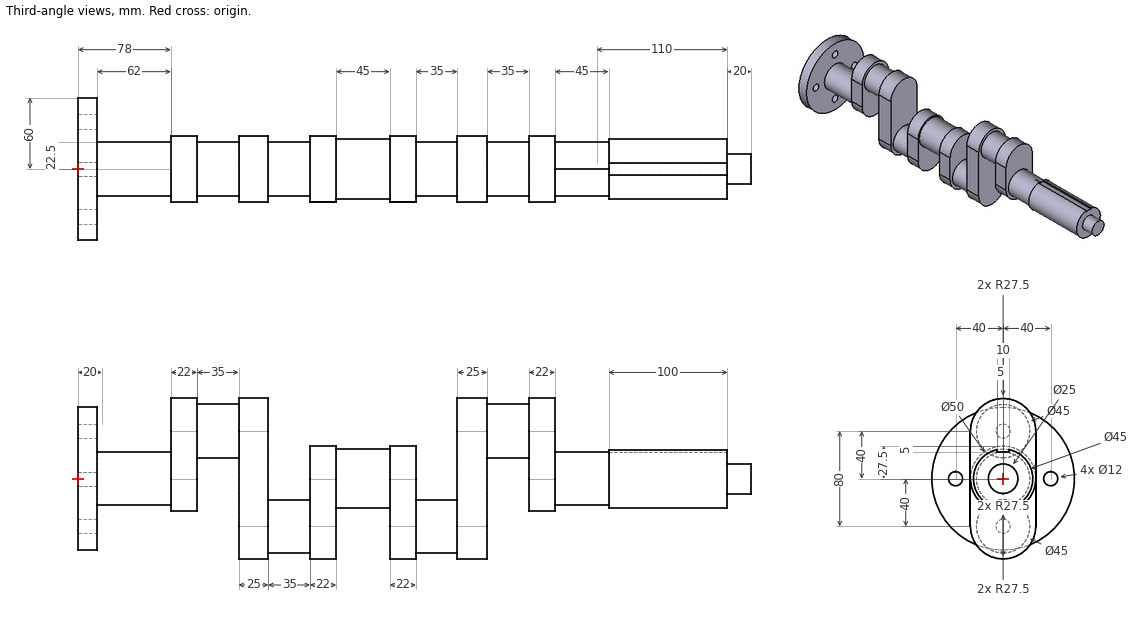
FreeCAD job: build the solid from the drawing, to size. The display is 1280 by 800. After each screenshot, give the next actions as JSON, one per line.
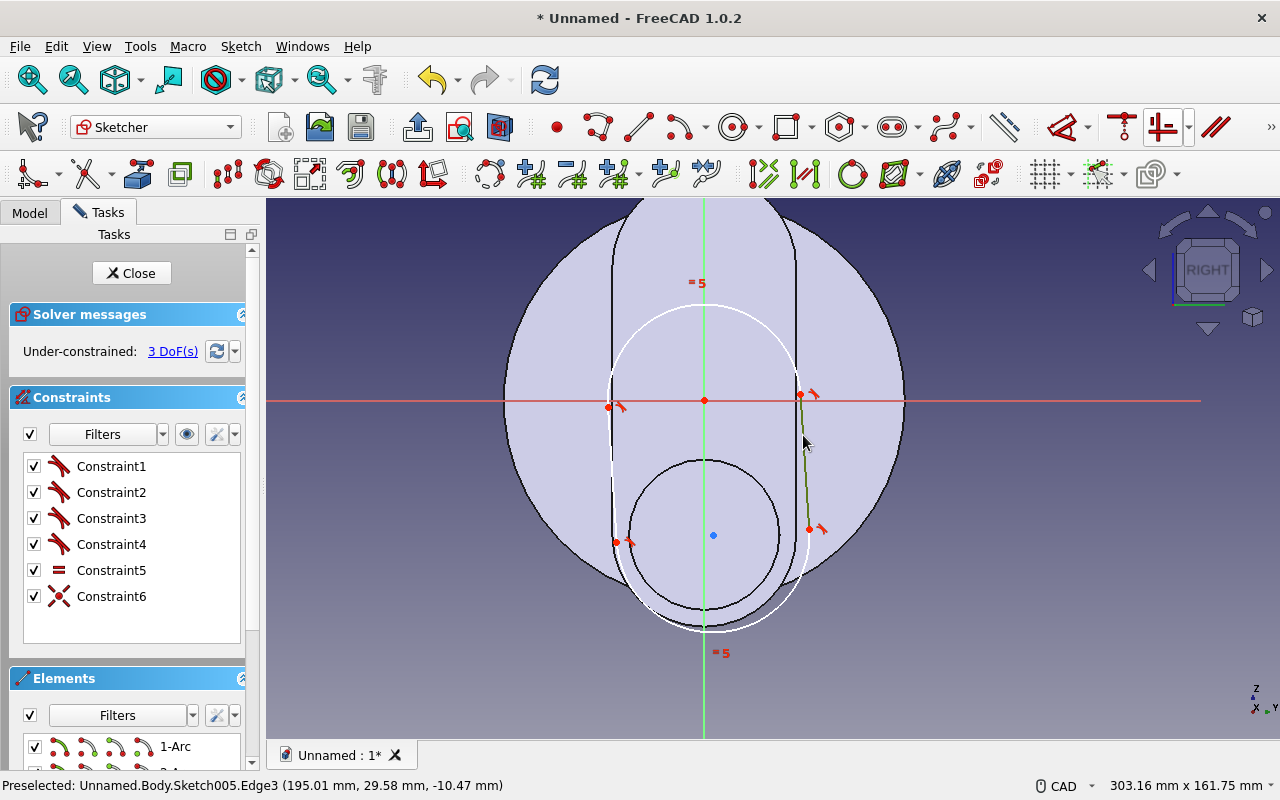
{"action": "left_click", "coordinate": [1188, 128]}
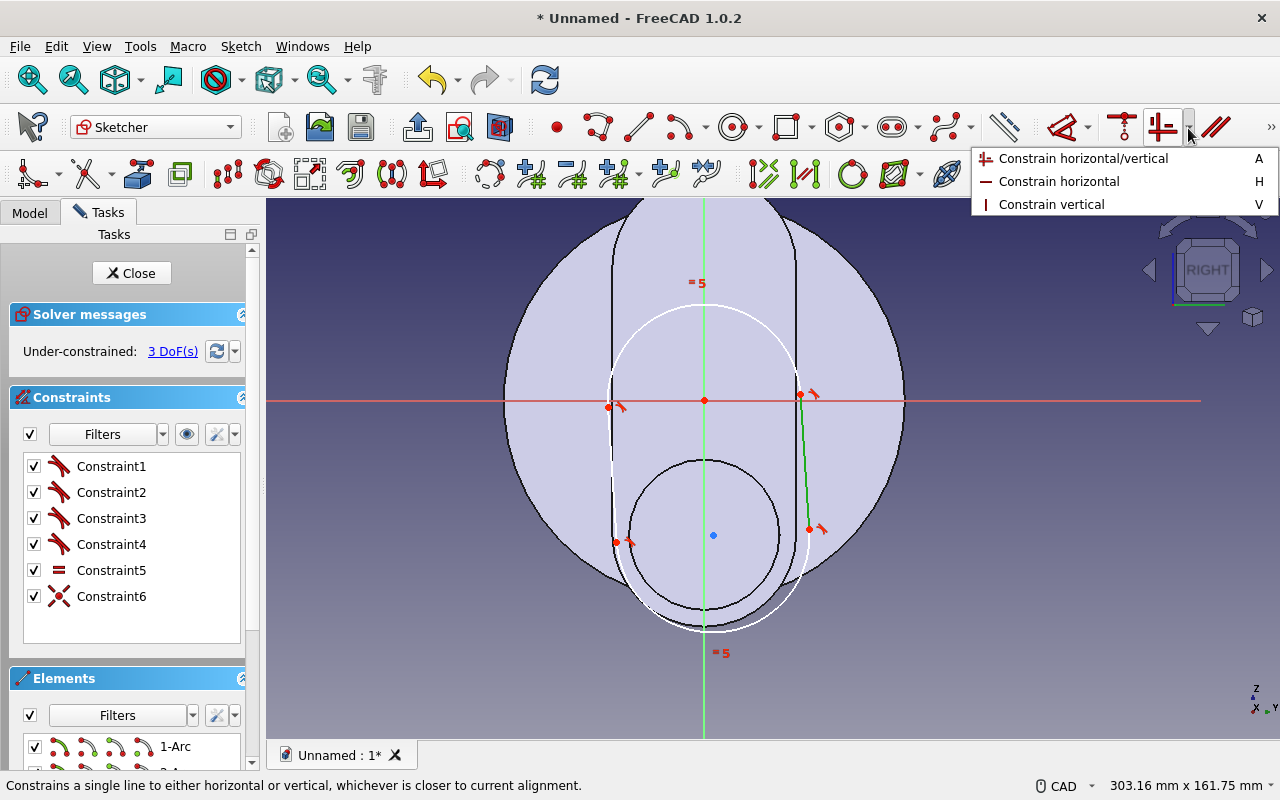
{"action": "left_click", "coordinate": [1125, 204]}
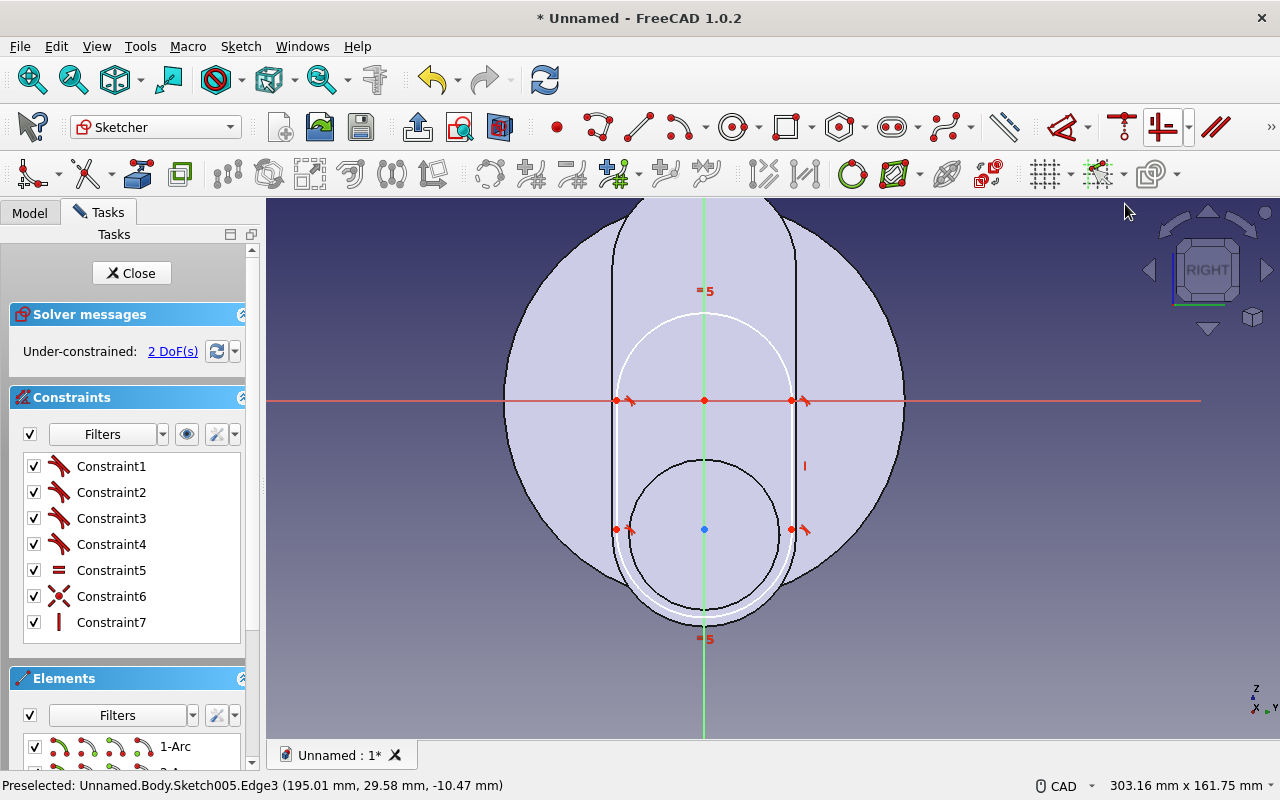
{"action": "left_click", "coordinate": [1062, 128]}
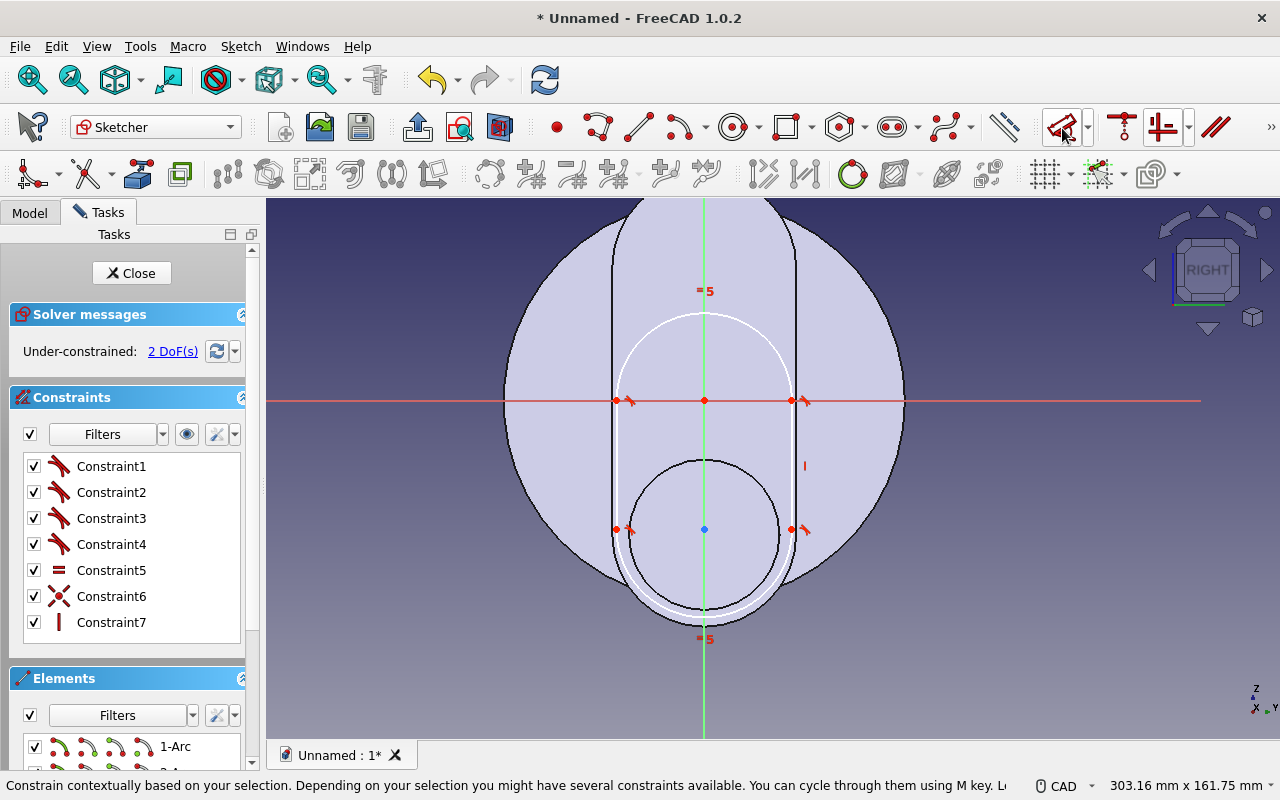
{"action": "left_click", "coordinate": [756, 330]}
{"action": "left_click", "coordinate": [775, 304]}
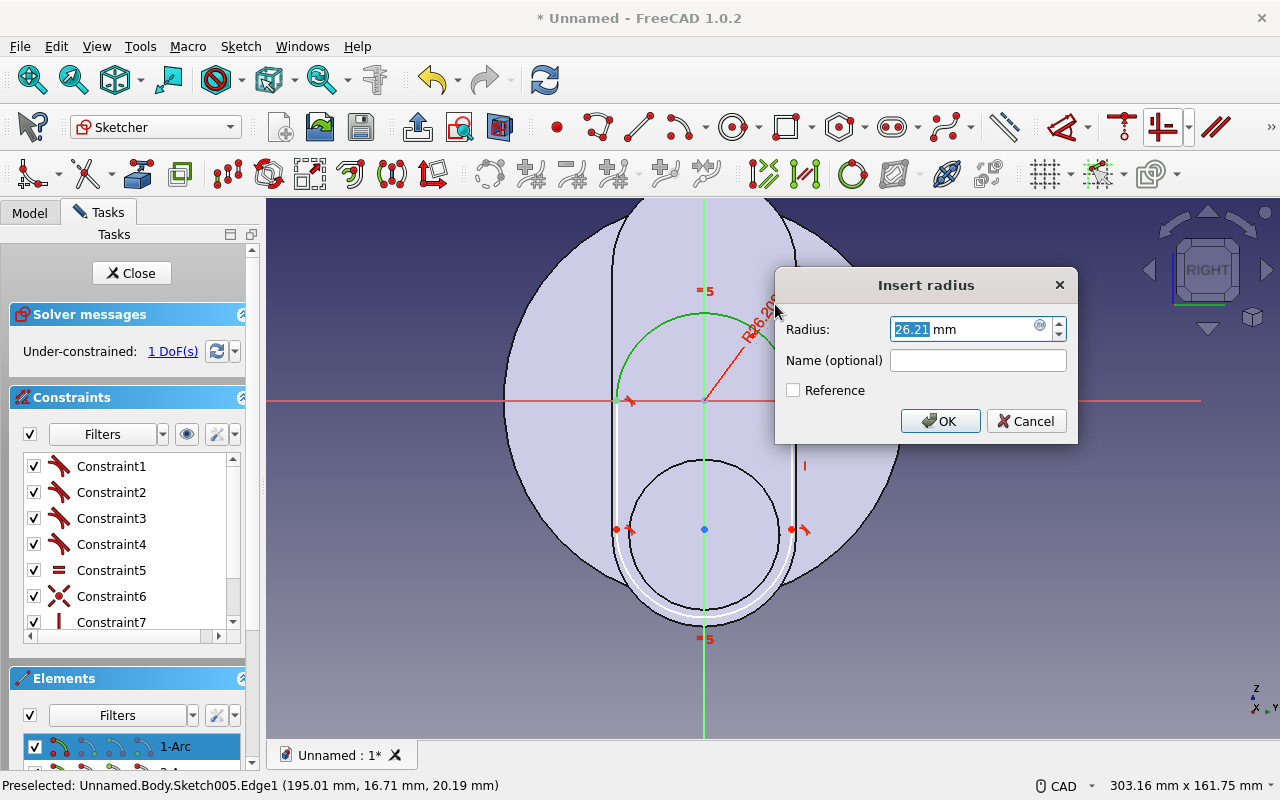
{"action": "type", "text": "27.5"}
{"action": "key", "text": "Return"}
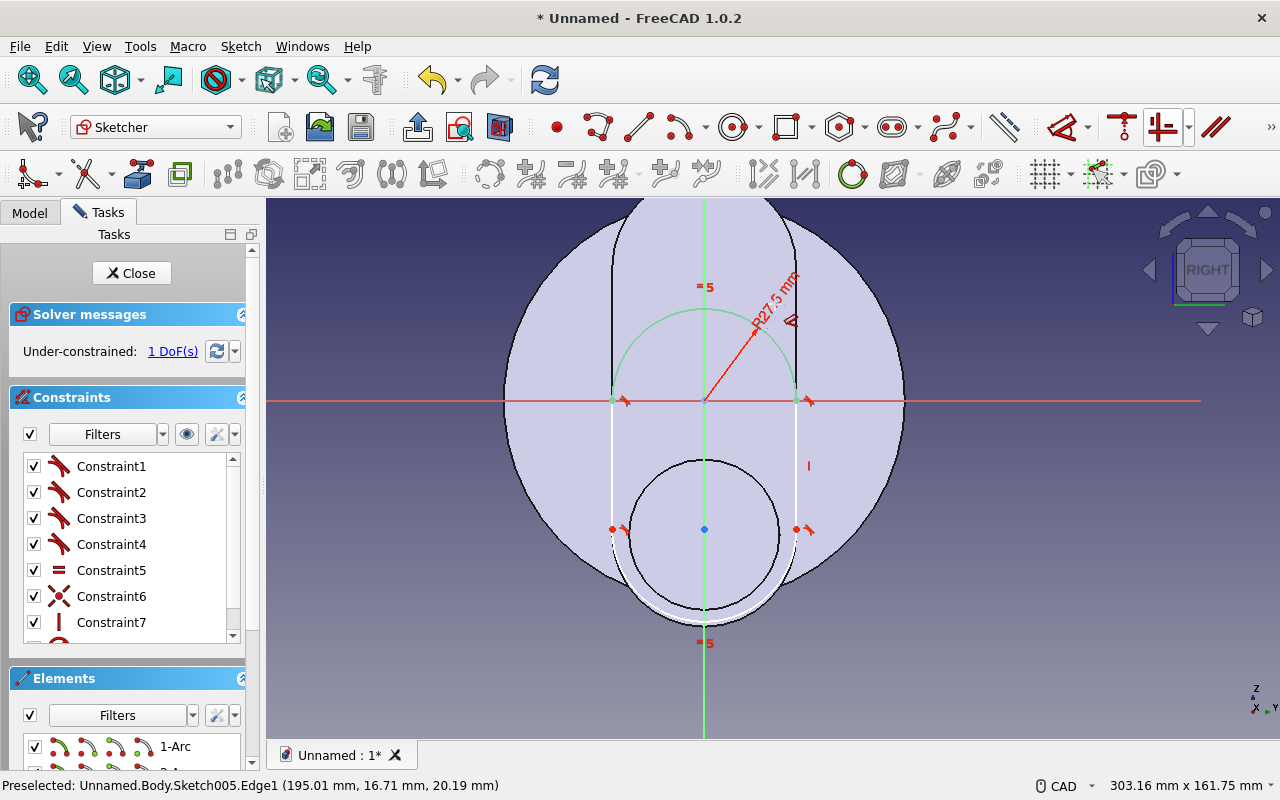
{"action": "left_click", "coordinate": [796, 440]}
{"action": "left_click", "coordinate": [830, 465]}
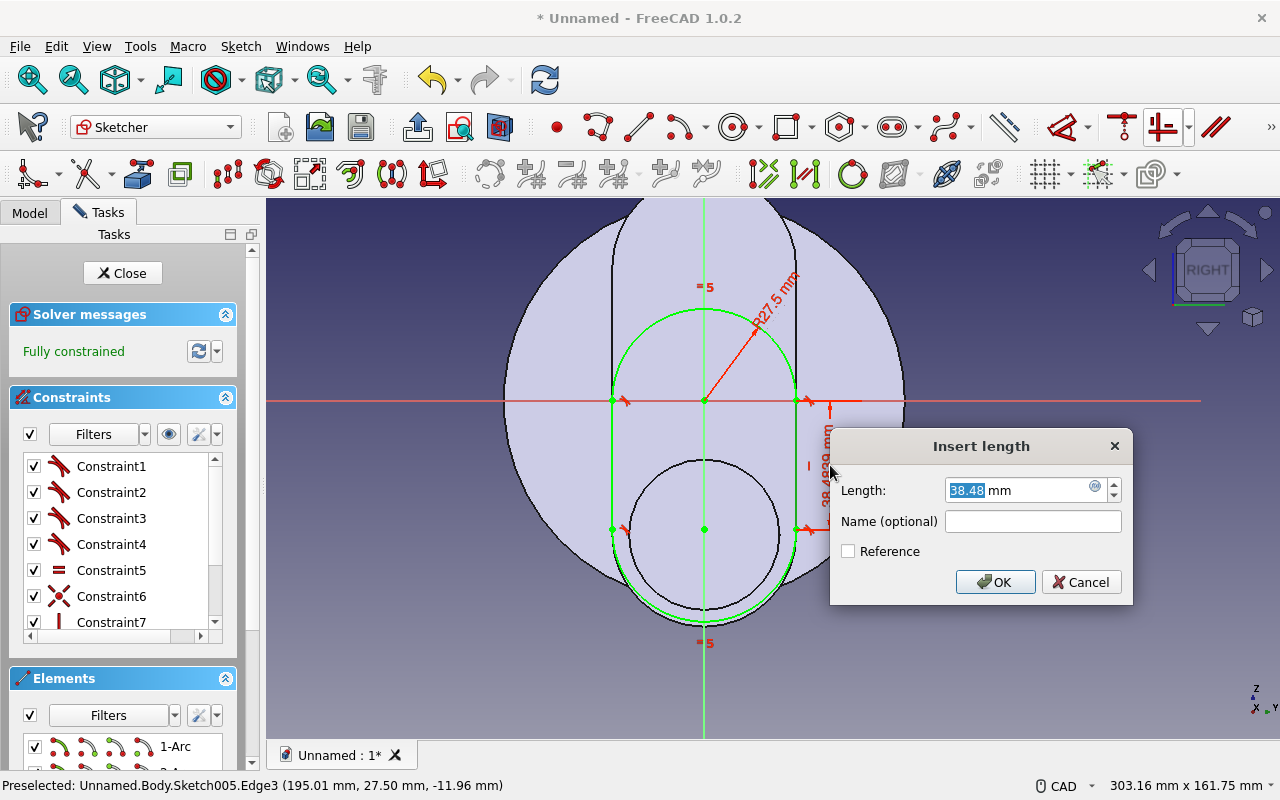
{"action": "type", "text": "40"}
{"action": "key", "text": "Return"}
{"action": "key", "text": "Escape"}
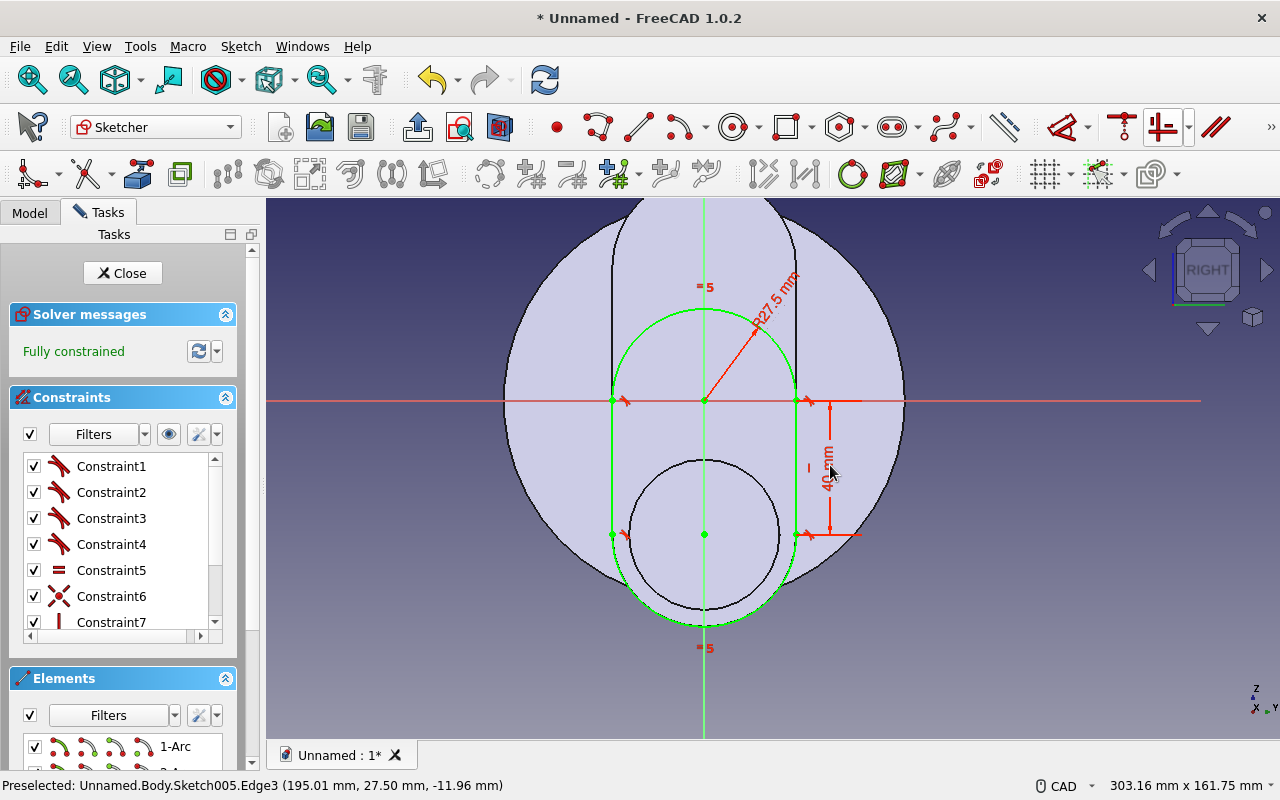
{"action": "left_click", "coordinate": [123, 273]}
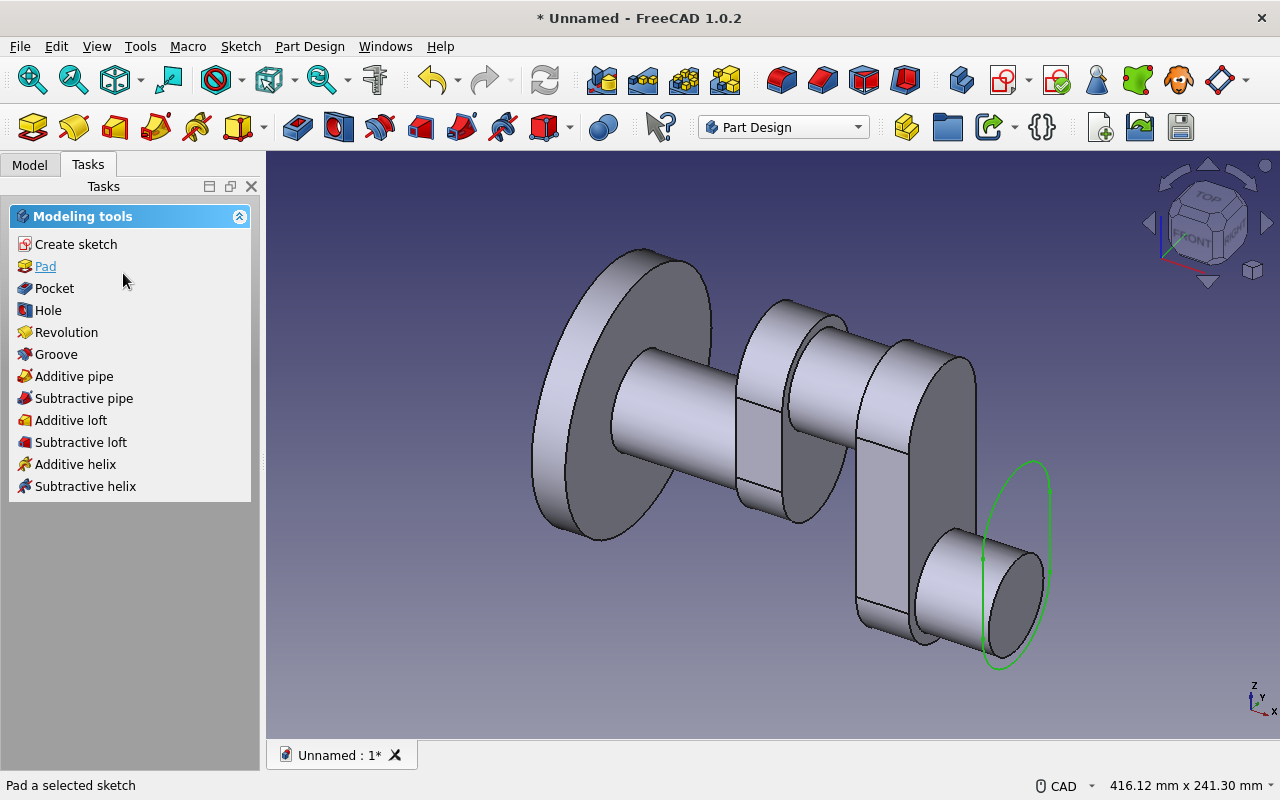
{"action": "left_click", "coordinate": [33, 128]}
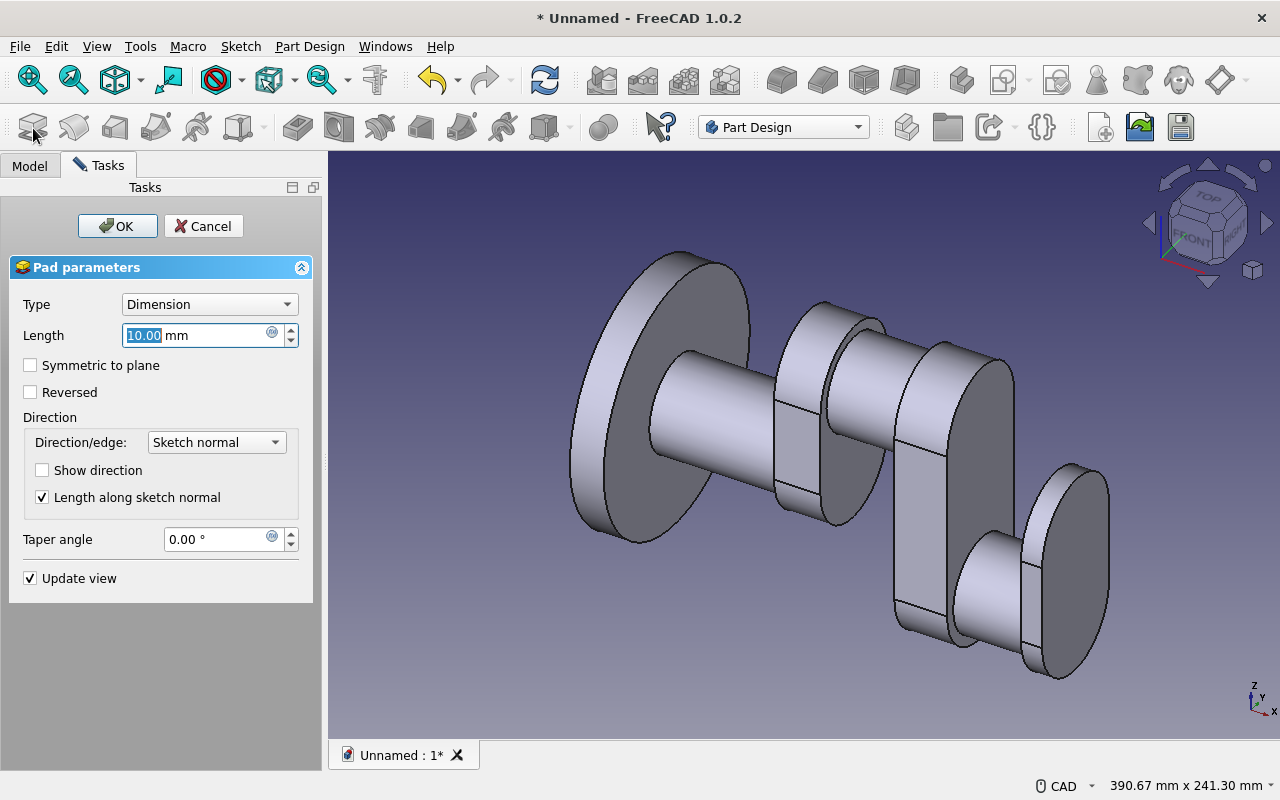
{"action": "type", "text": "22"}
{"action": "key", "text": "Tab"}